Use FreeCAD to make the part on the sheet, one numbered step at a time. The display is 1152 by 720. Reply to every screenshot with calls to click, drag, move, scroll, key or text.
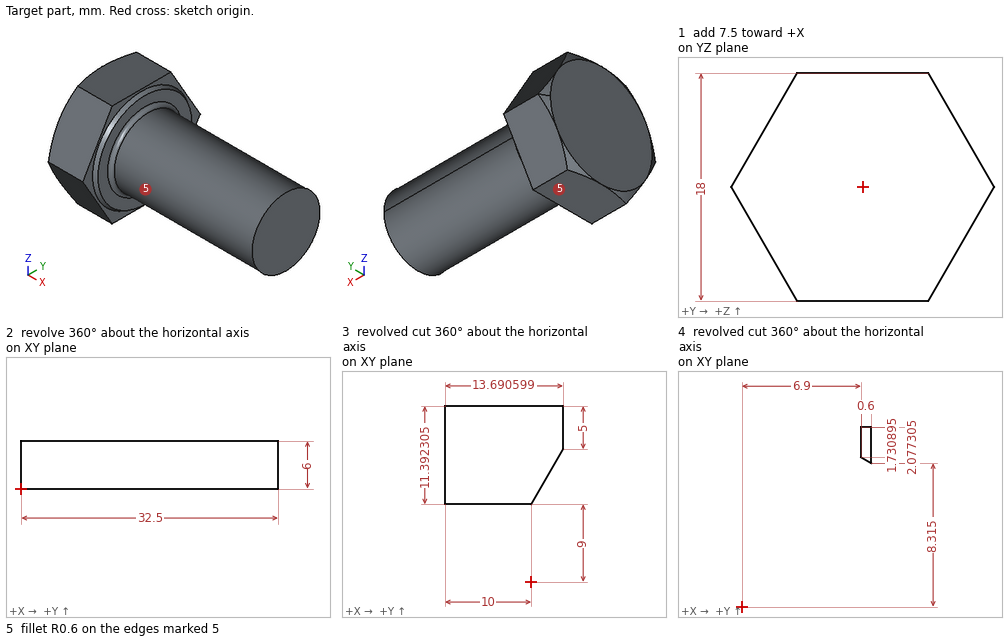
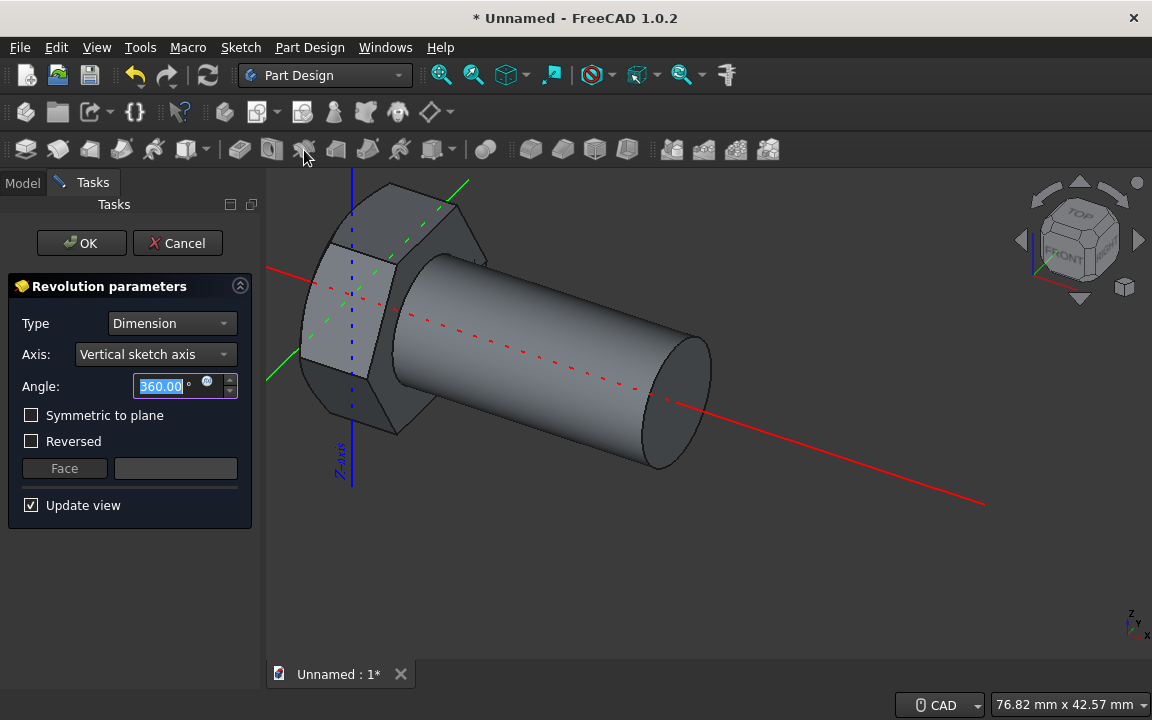
click(156, 354)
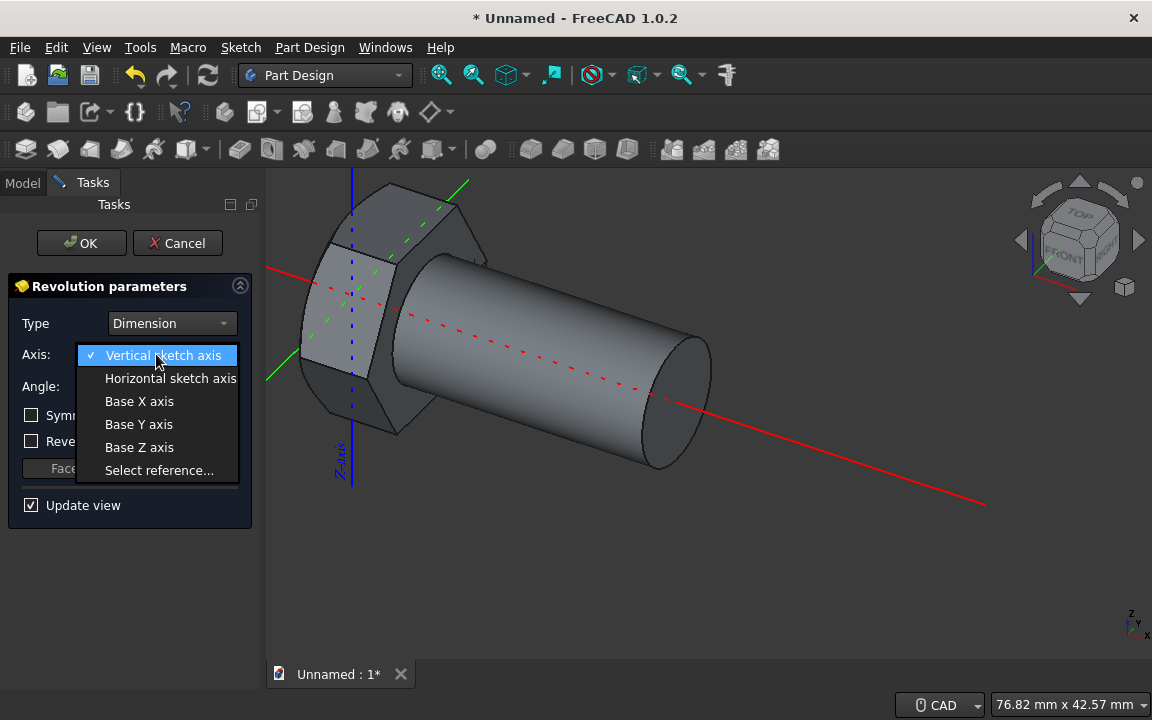
click(156, 378)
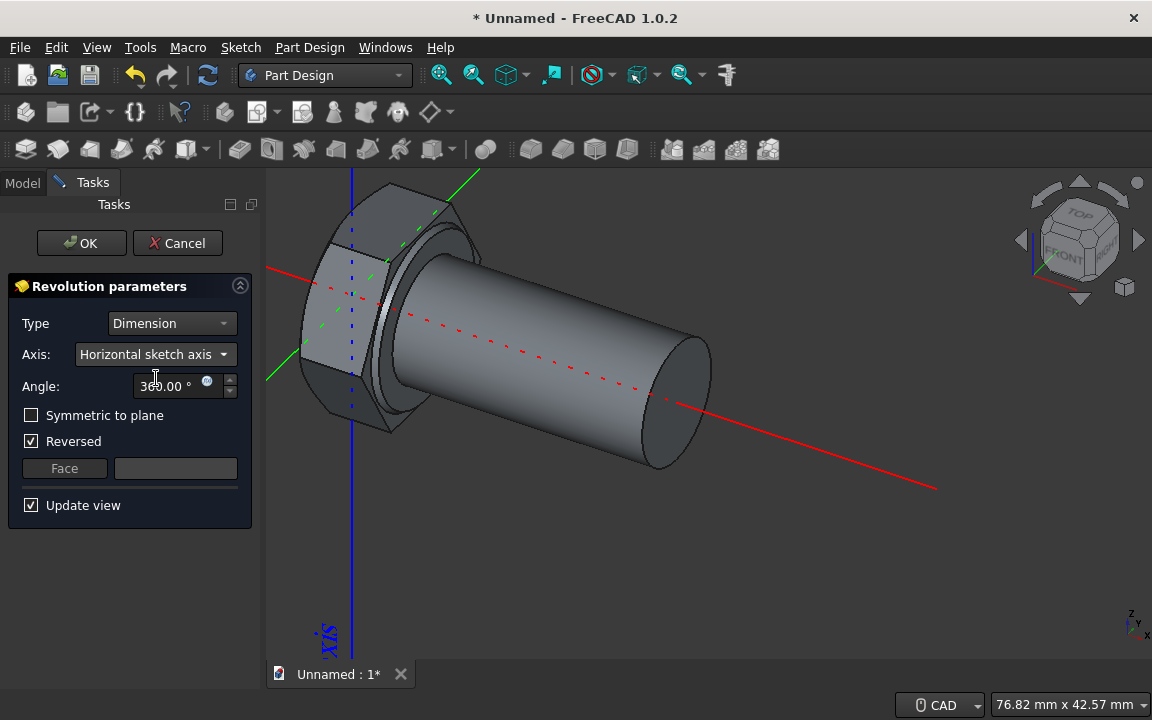
click(82, 243)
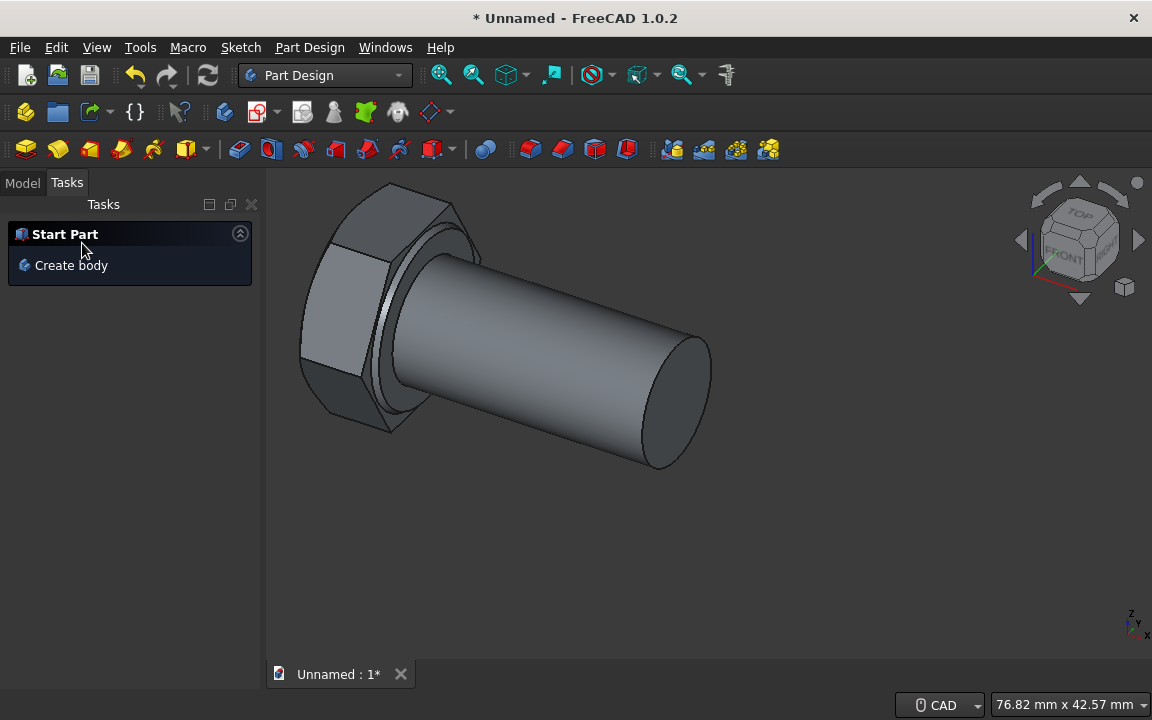
click(442, 76)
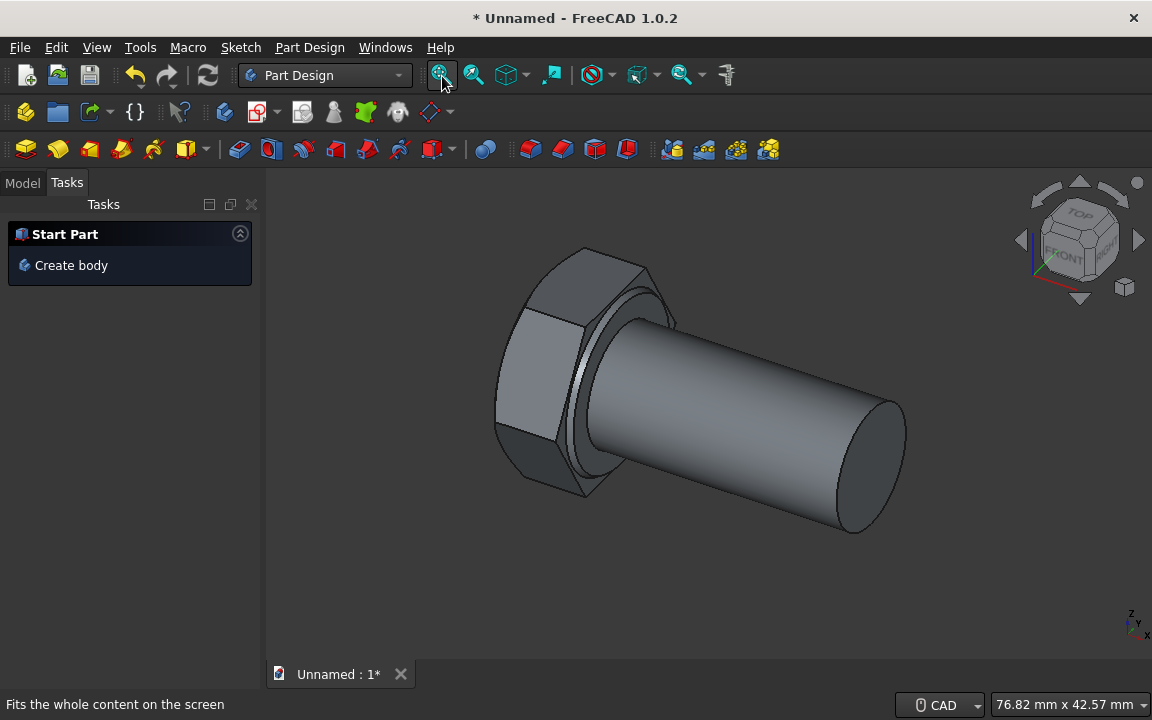
key(0)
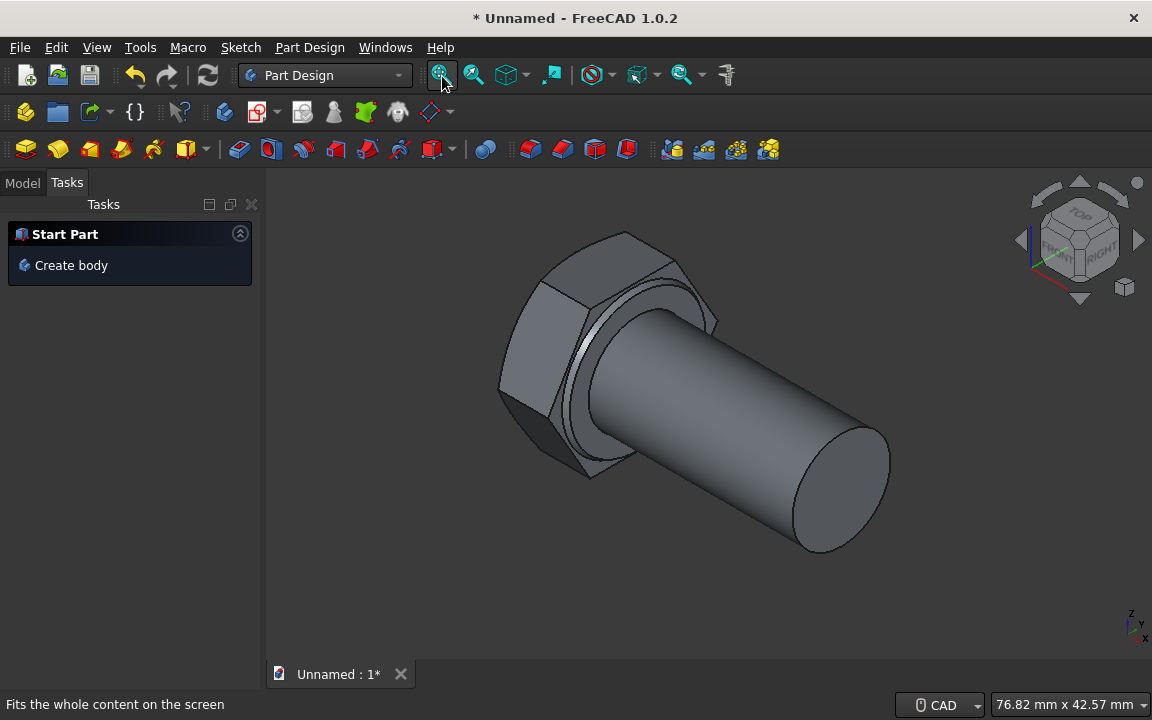
key(2)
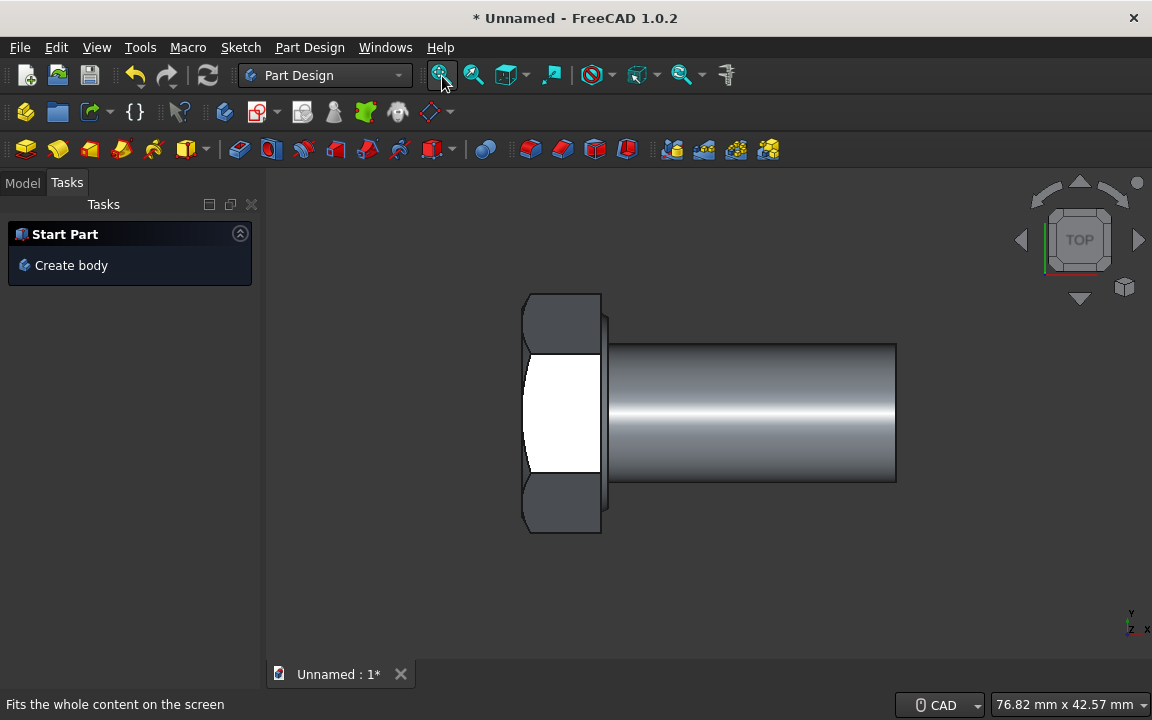
key(1)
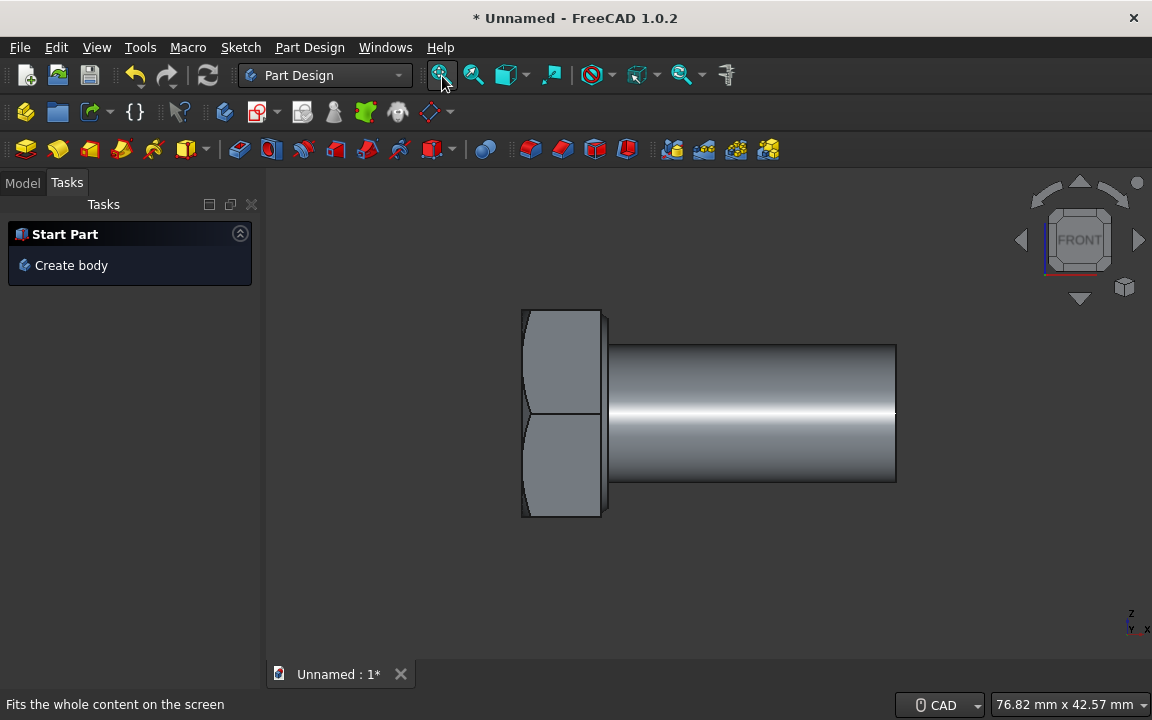
click(442, 76)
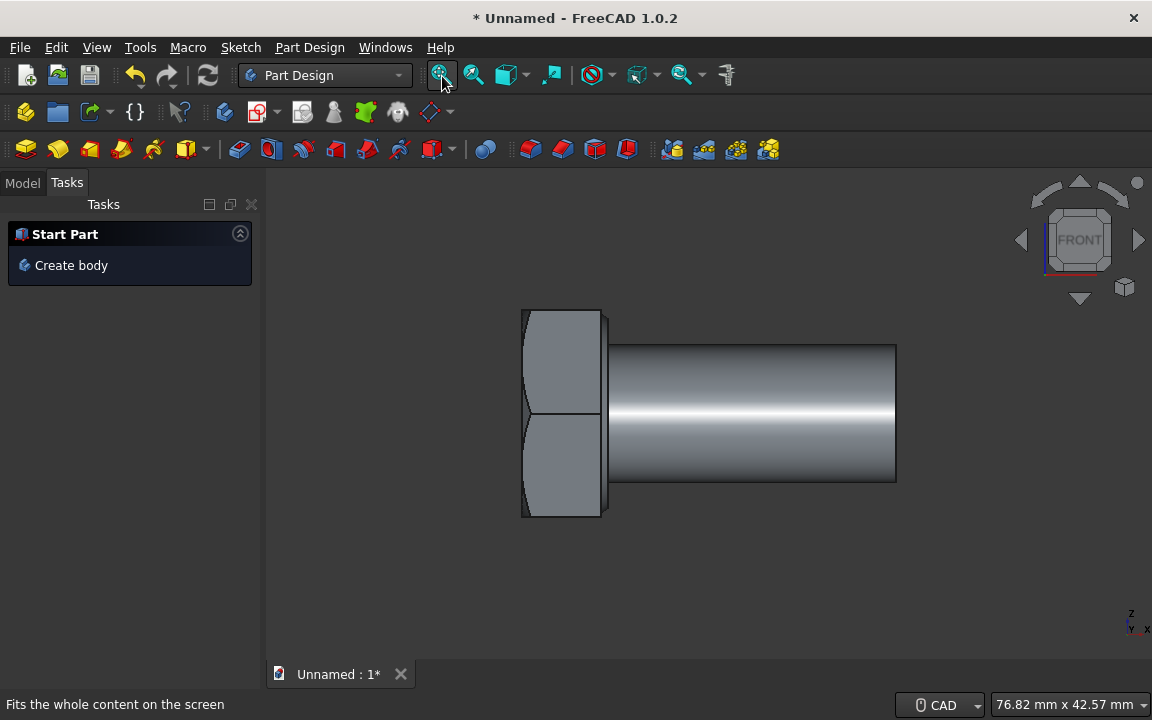
key(3)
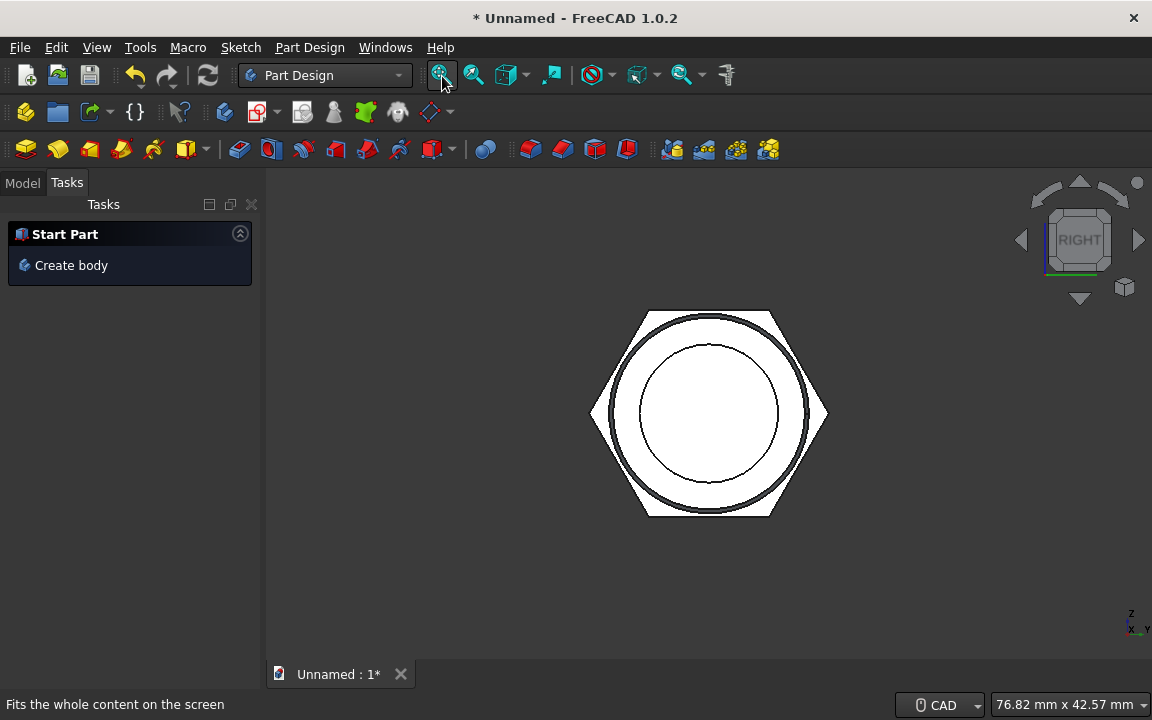
click(442, 76)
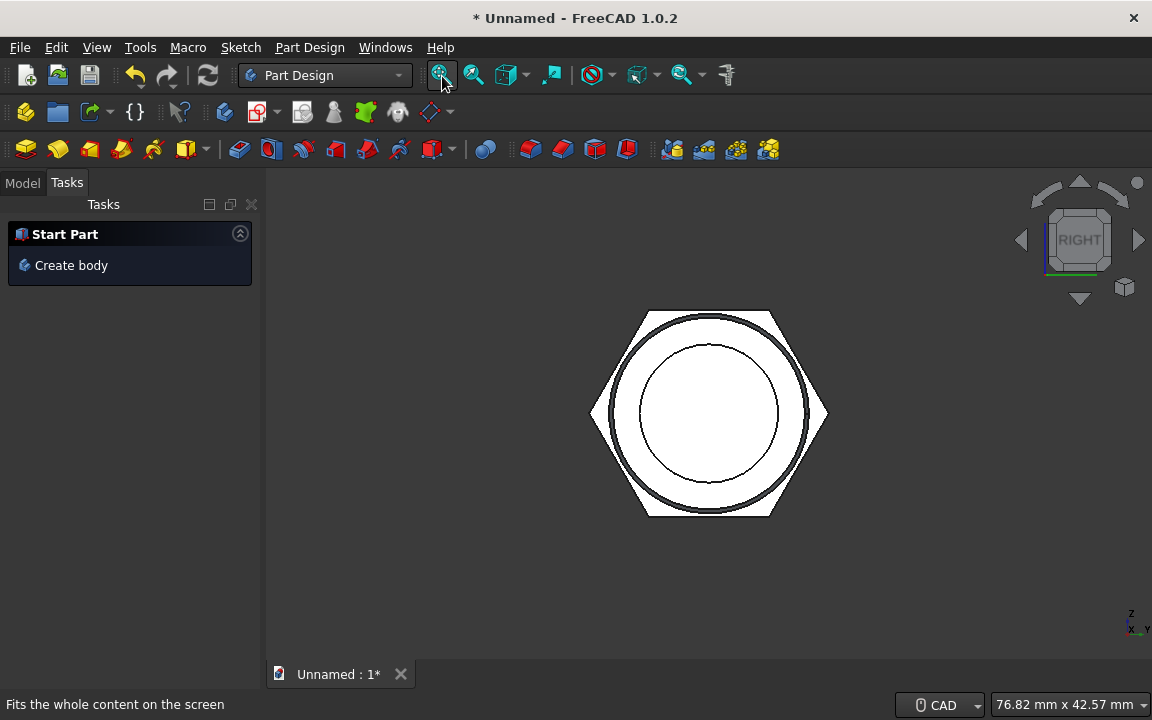
key(5)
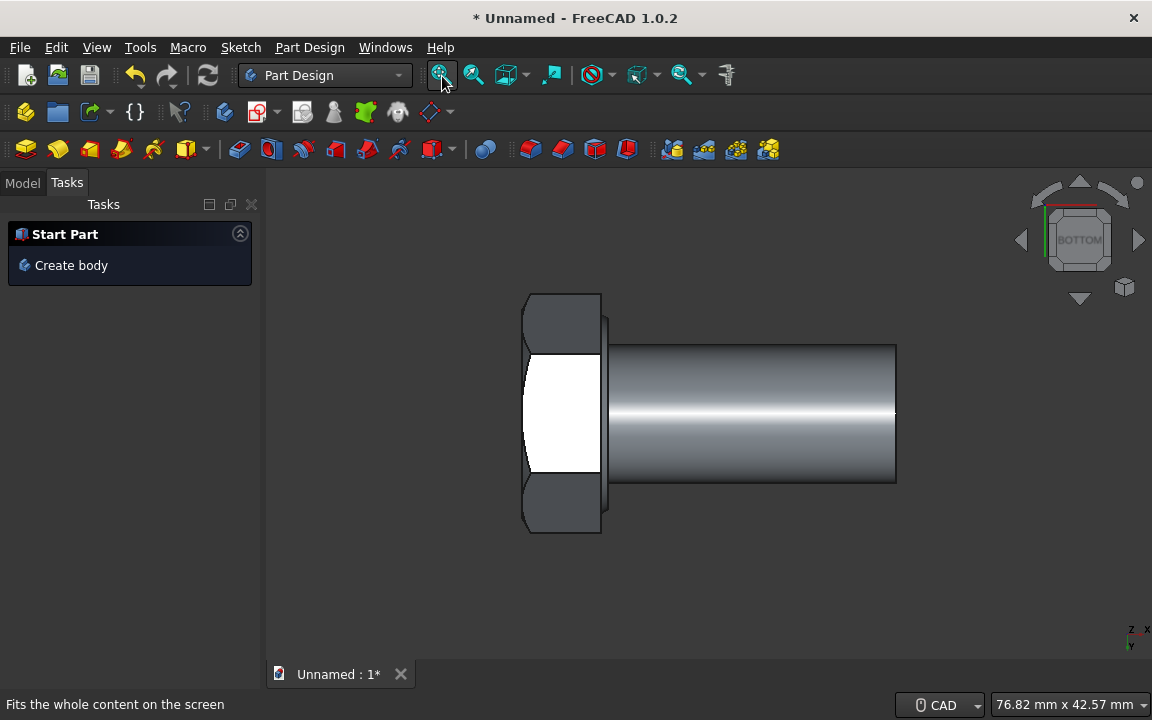
key(4)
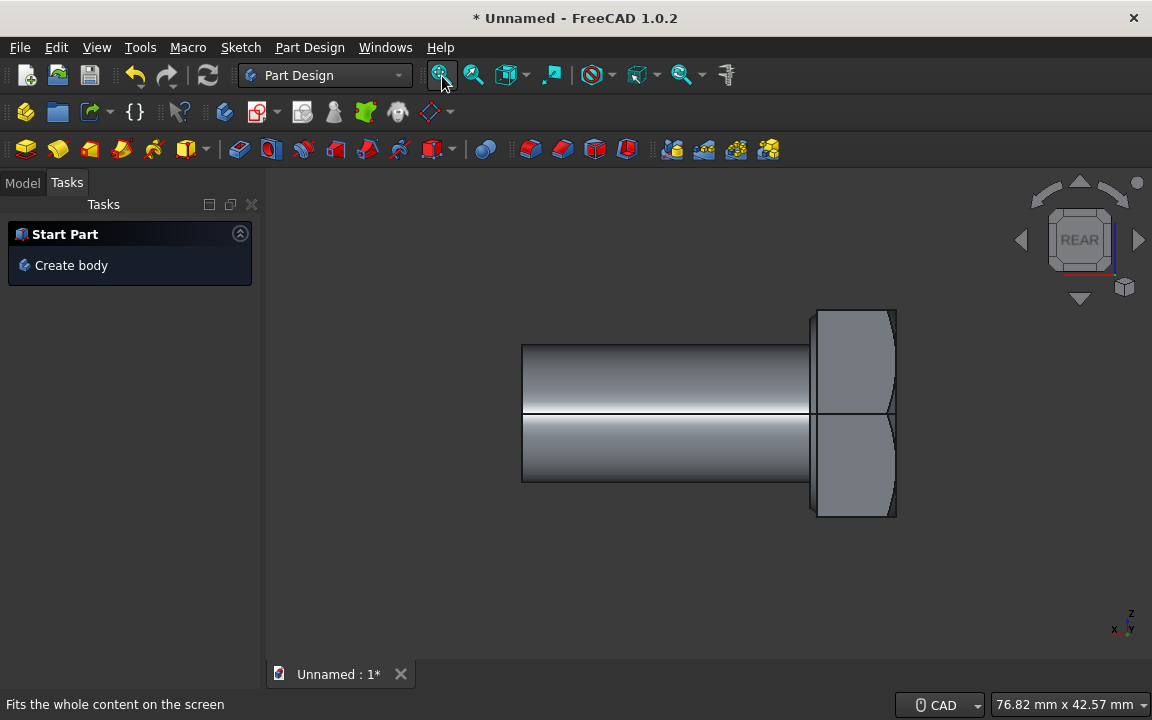
click(442, 76)